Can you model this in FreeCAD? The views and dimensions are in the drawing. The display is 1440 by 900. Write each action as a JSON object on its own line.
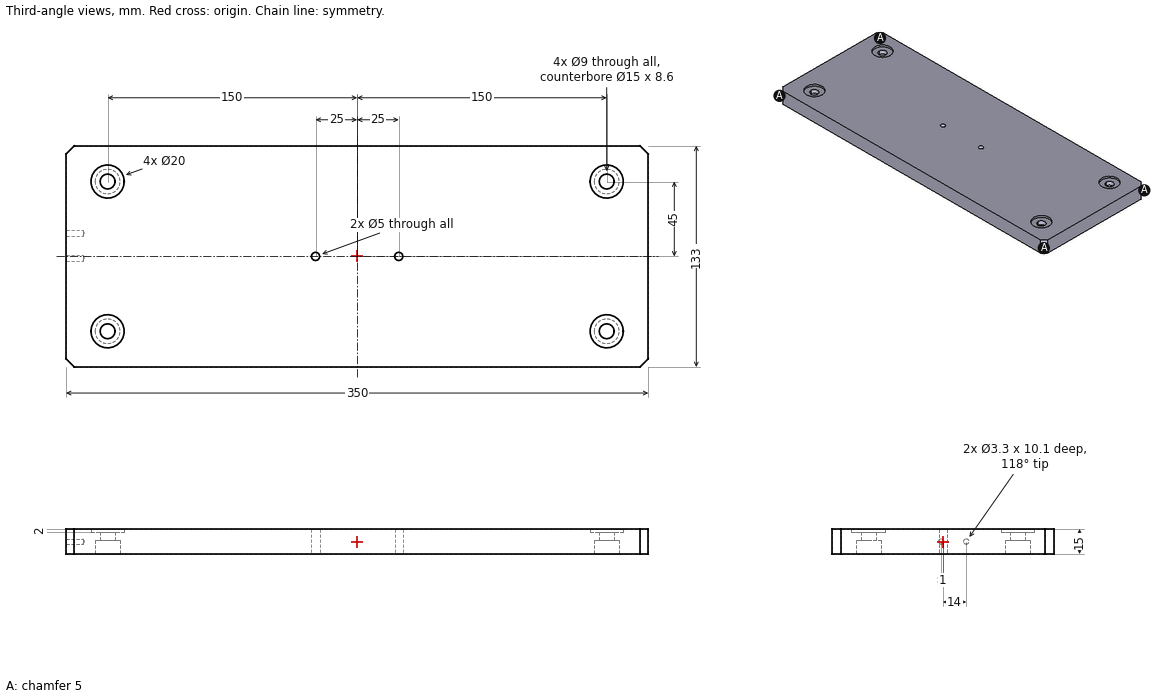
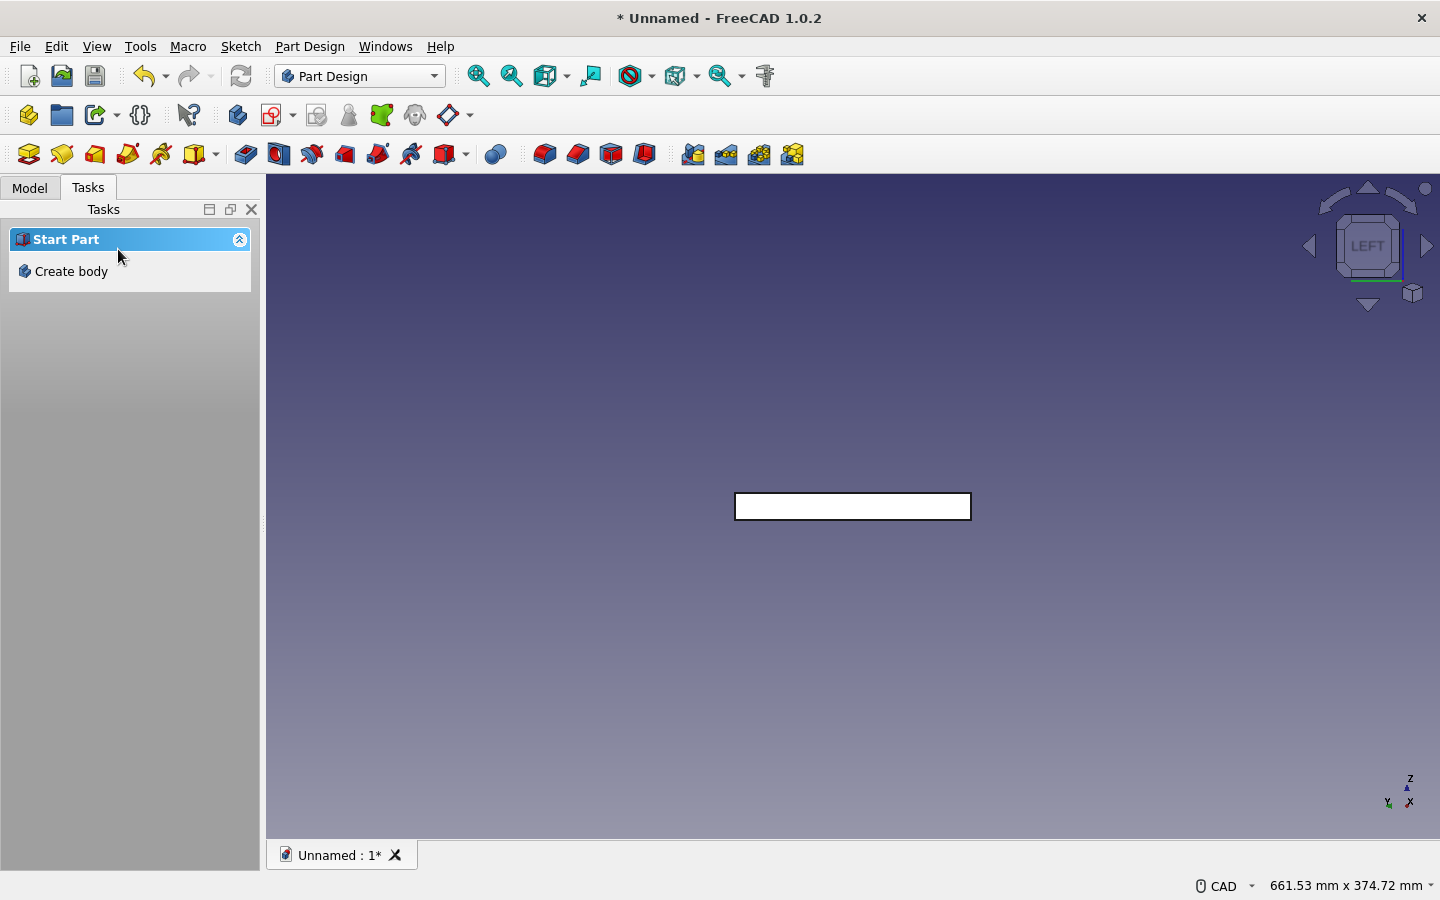
{"action": "left_click", "coordinate": [752, 505]}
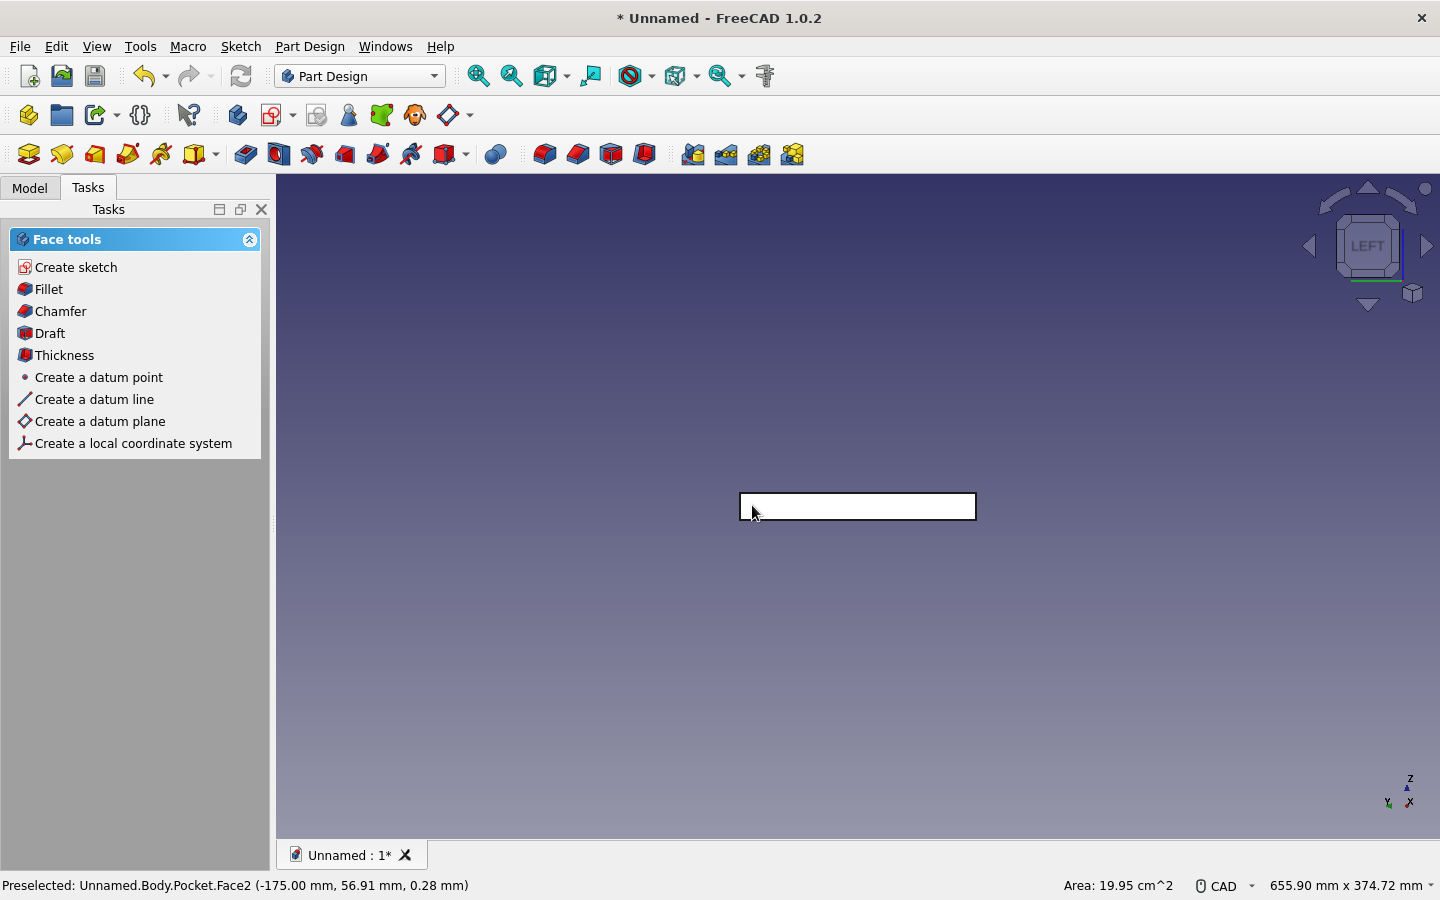
{"action": "left_click", "coordinate": [270, 116]}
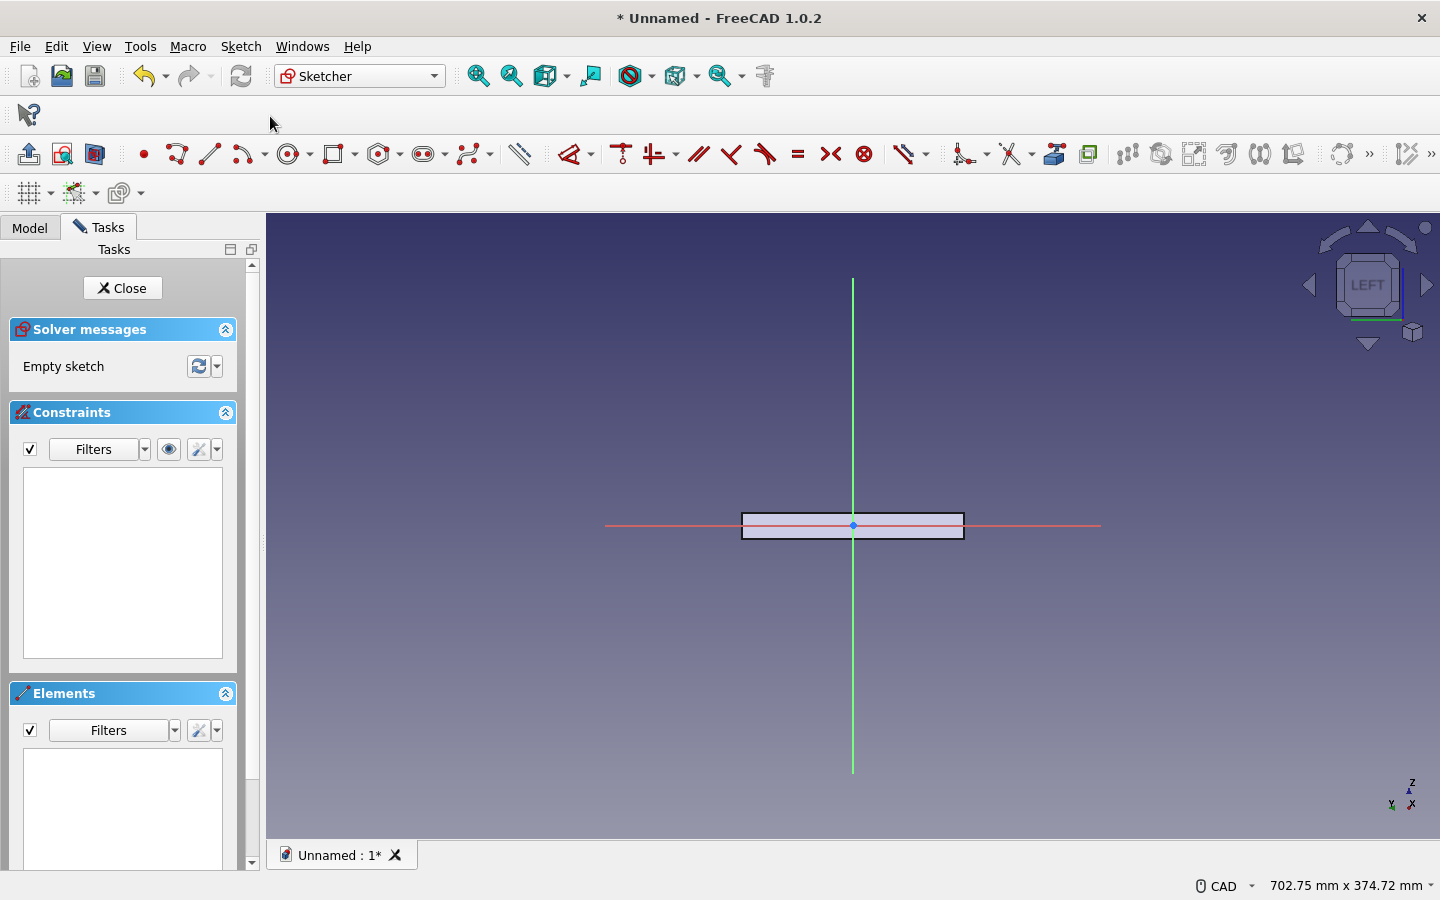
{"action": "scroll", "coordinate": [845, 526], "scroll_direction": "up", "scroll_amount": 15}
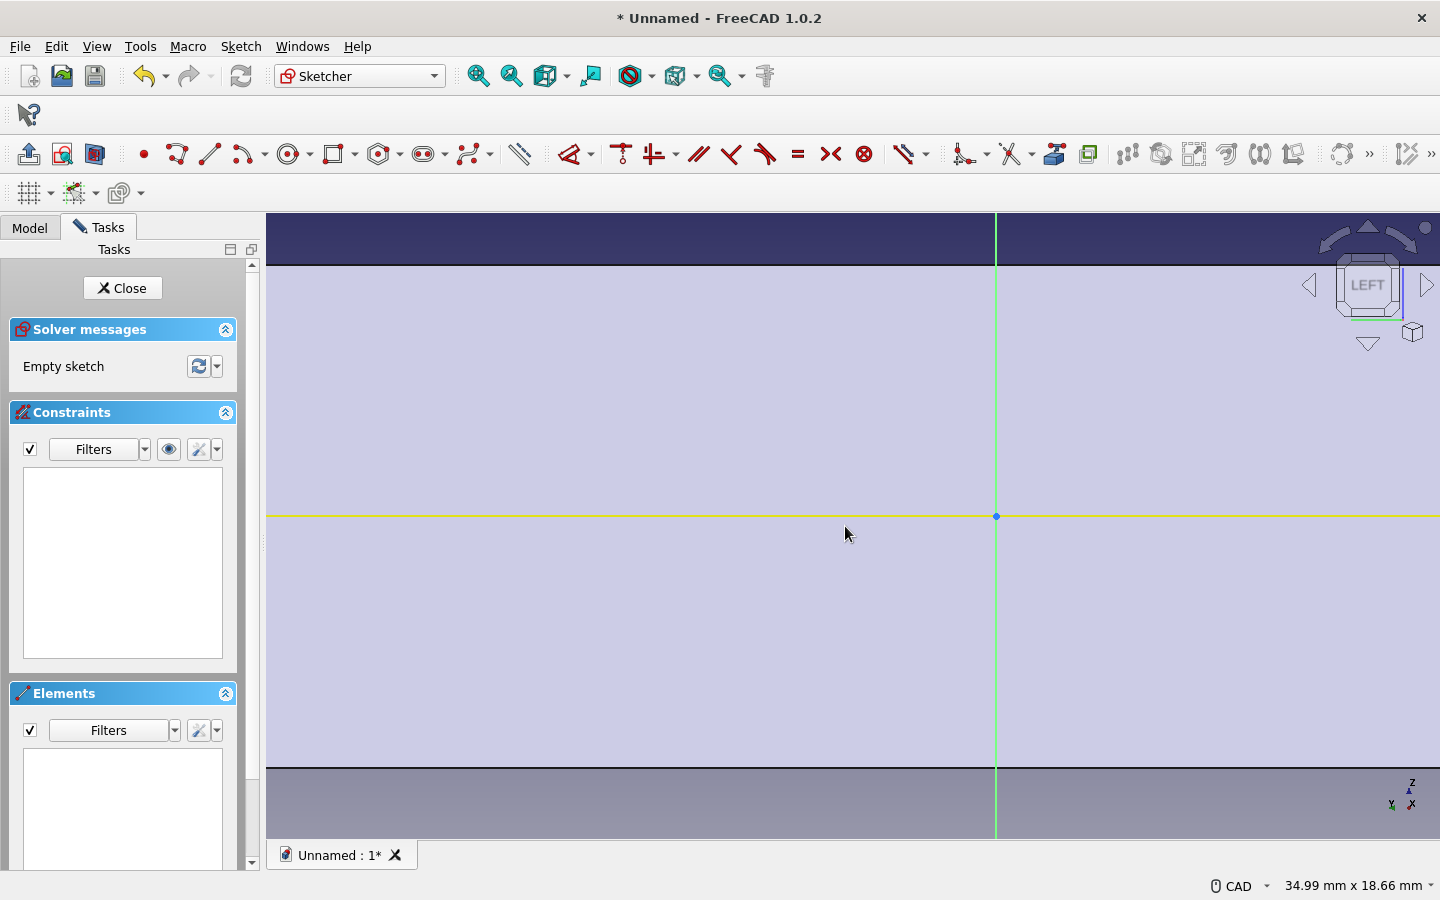
{"action": "key", "text": "g c"}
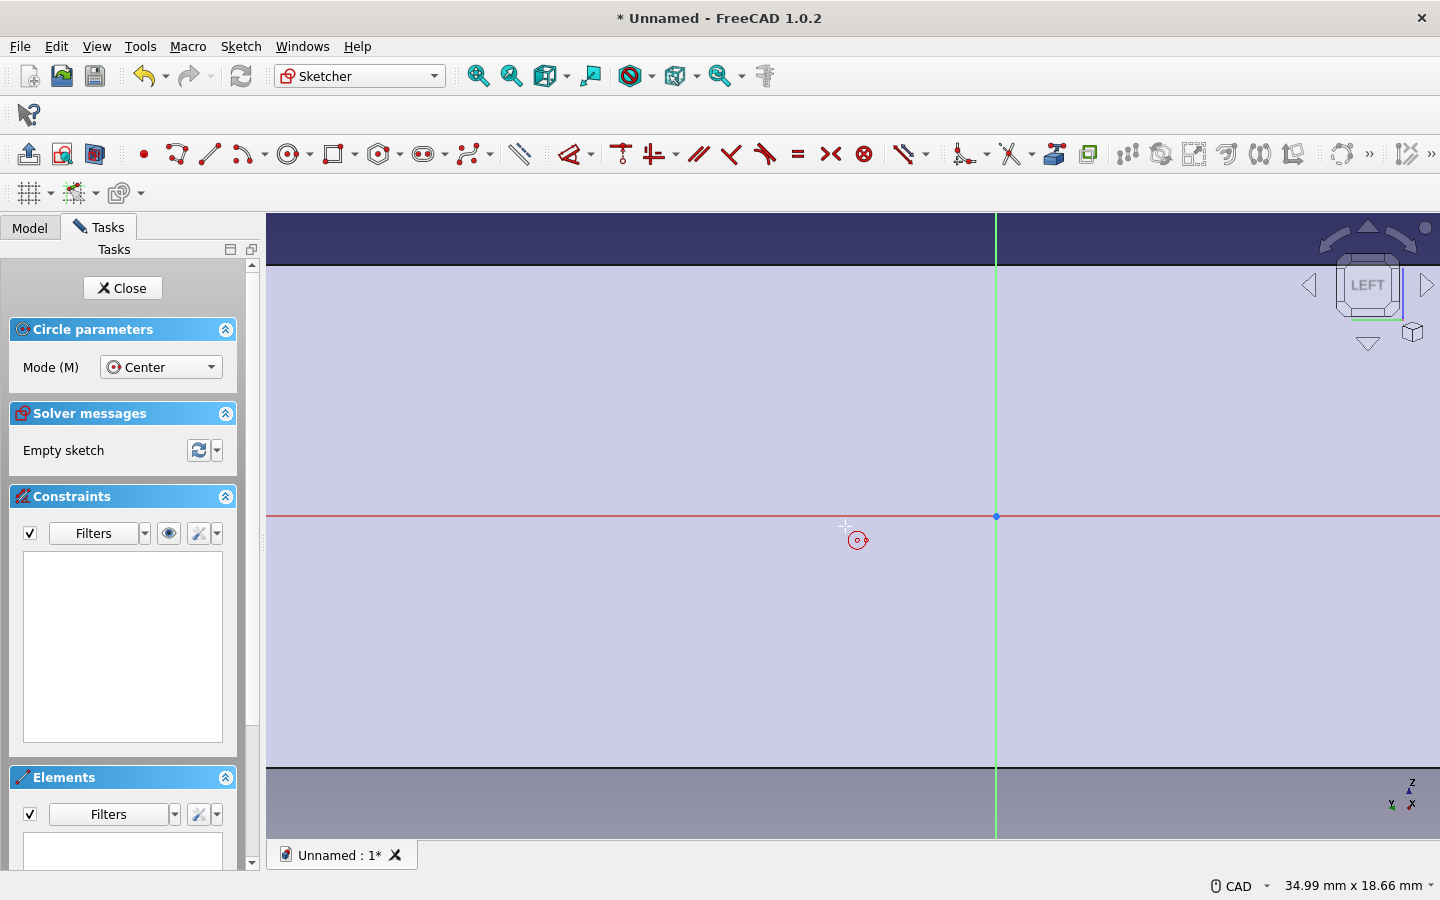
{"action": "left_click", "coordinate": [526, 516]}
{"action": "mouse_move", "coordinate": [566, 477]}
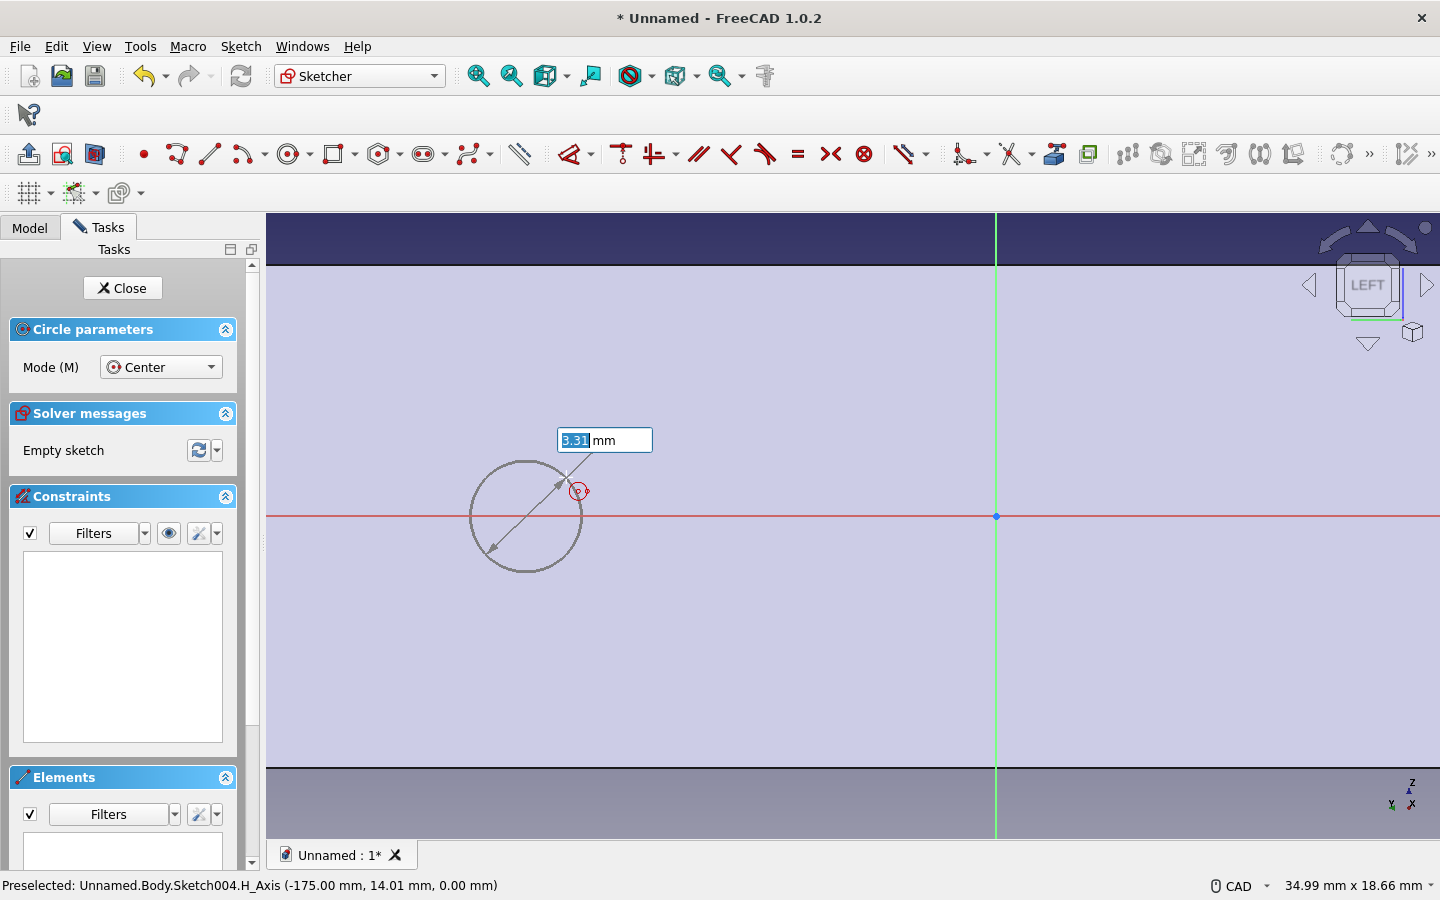
{"action": "type", "text": "3.3"}
{"action": "key", "text": "Return"}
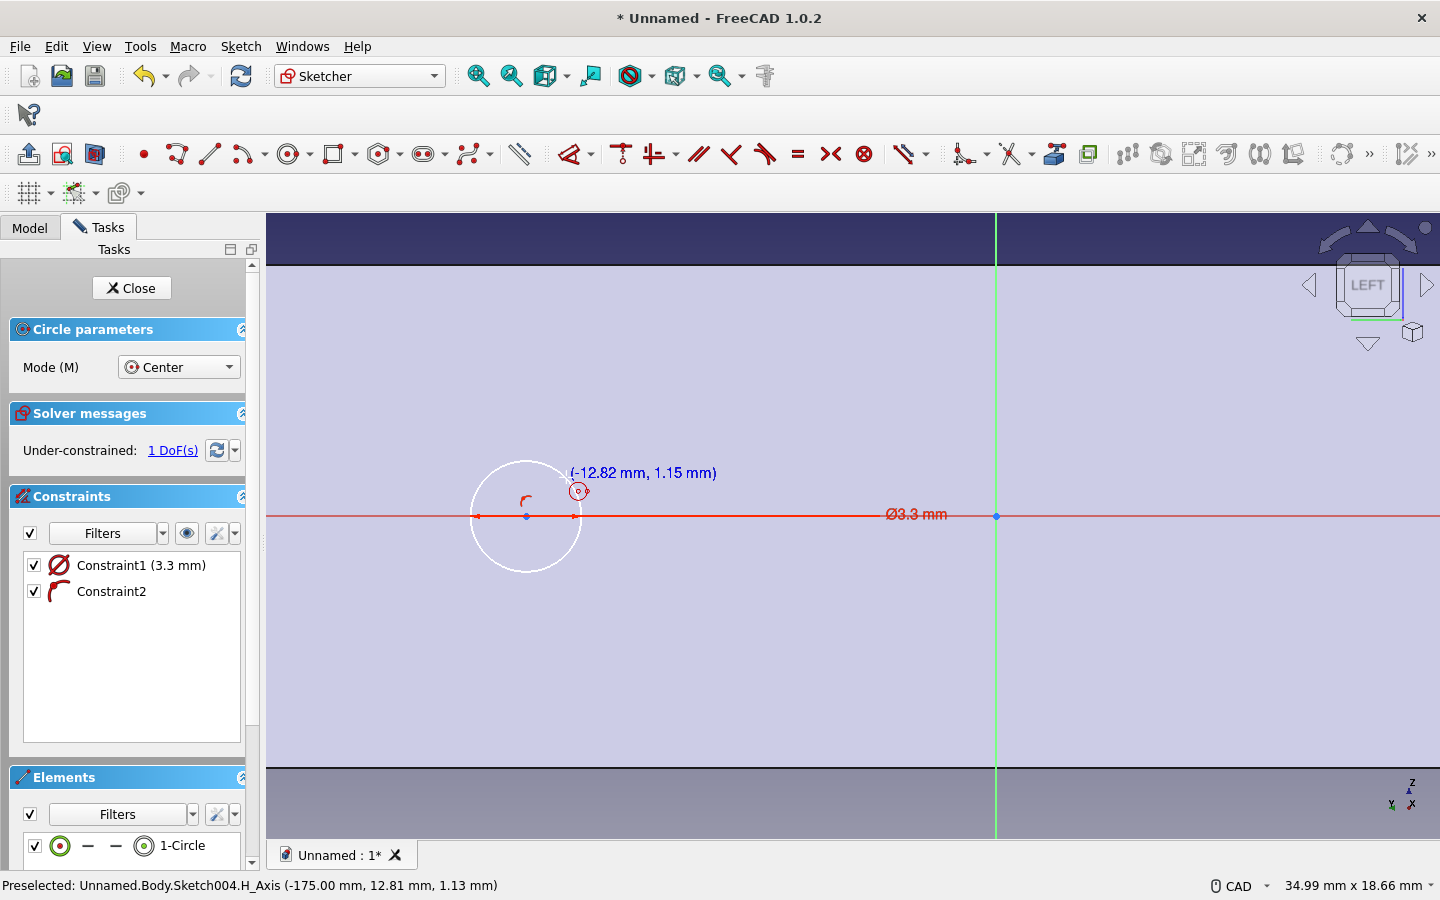
{"action": "left_click", "coordinate": [1030, 516]}
{"action": "mouse_move", "coordinate": [1069, 477]}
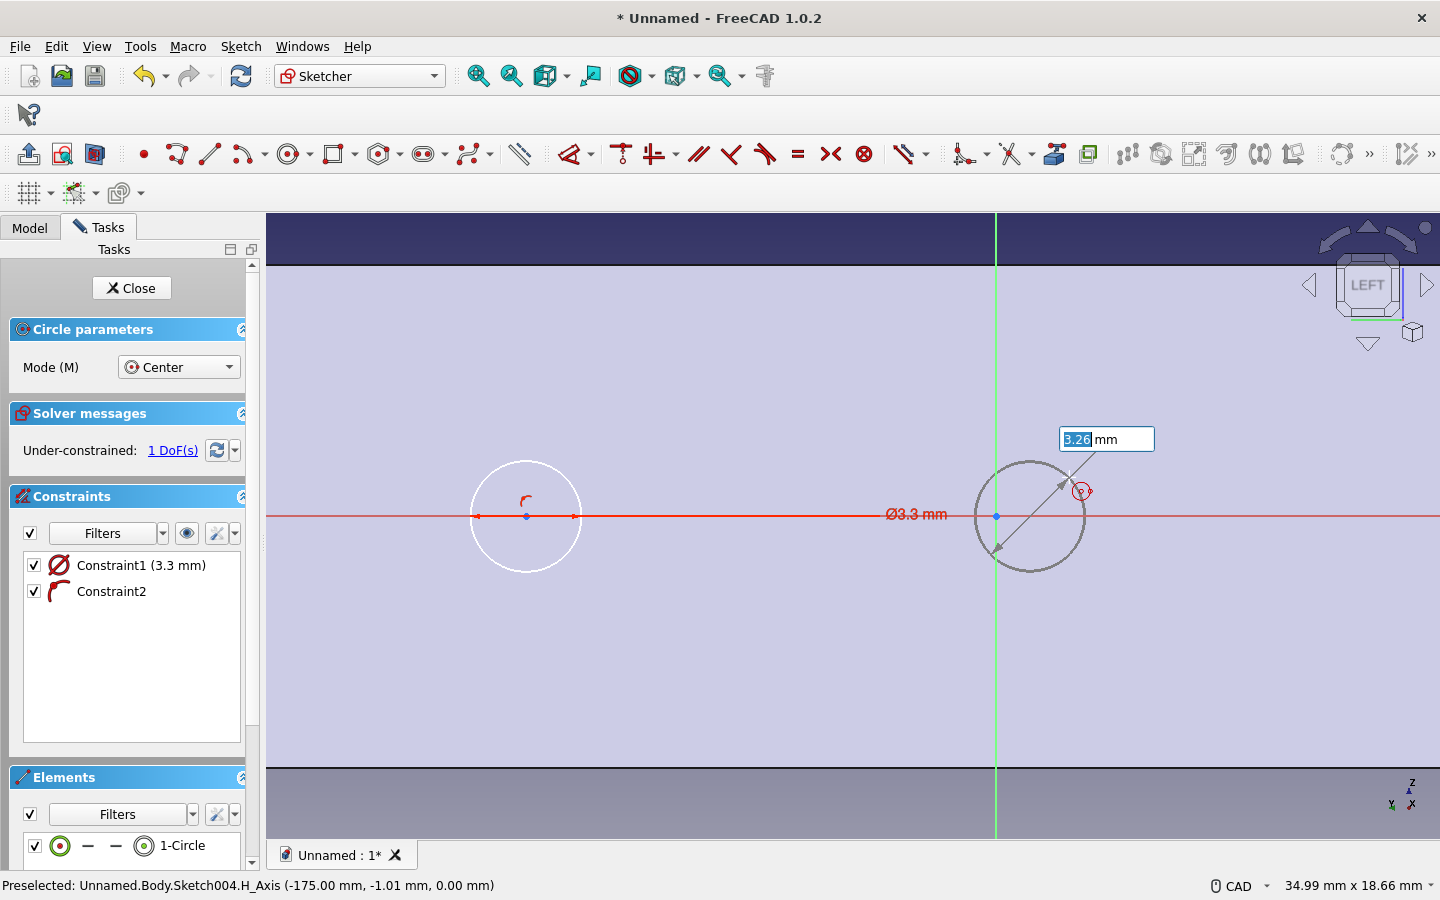
{"action": "type", "text": "3.3"}
{"action": "key", "text": "Return"}
{"action": "key", "text": "Escape"}